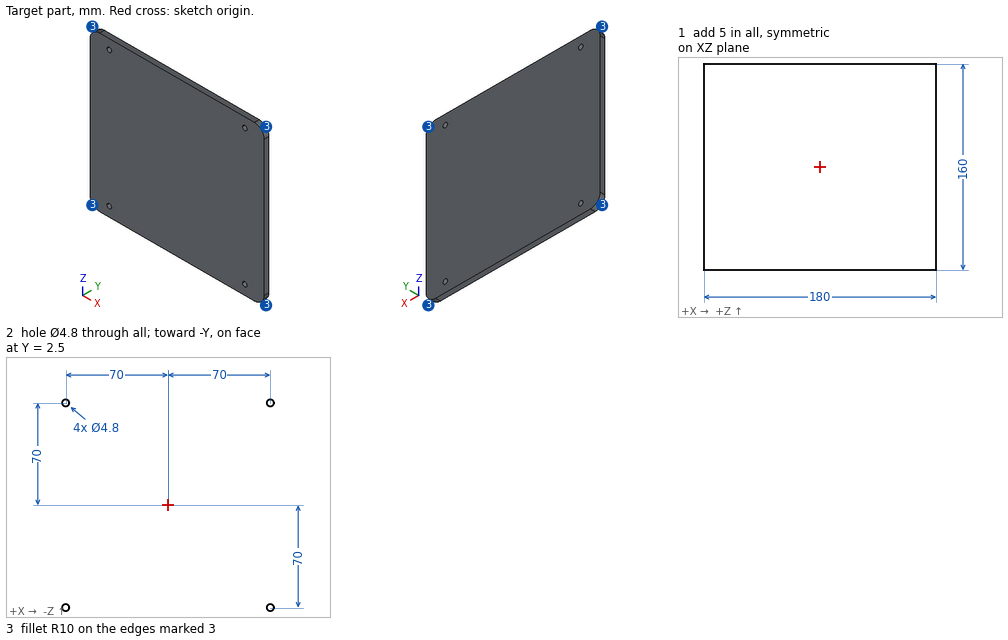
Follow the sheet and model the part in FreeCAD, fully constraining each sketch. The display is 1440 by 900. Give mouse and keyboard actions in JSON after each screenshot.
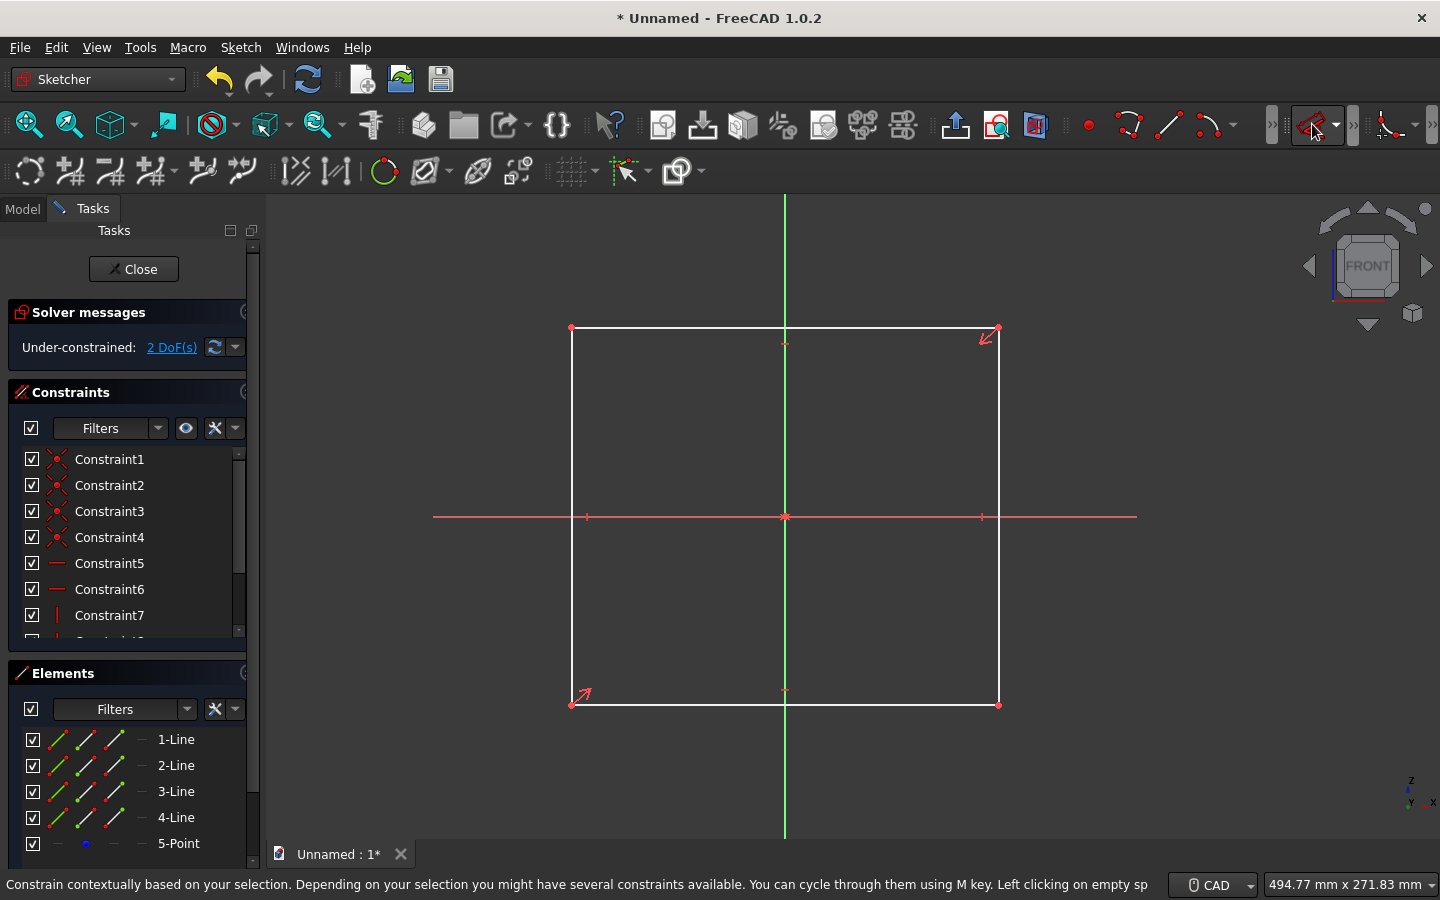
{"action": "left_click", "coordinate": [700, 705]}
{"action": "left_click", "coordinate": [687, 739]}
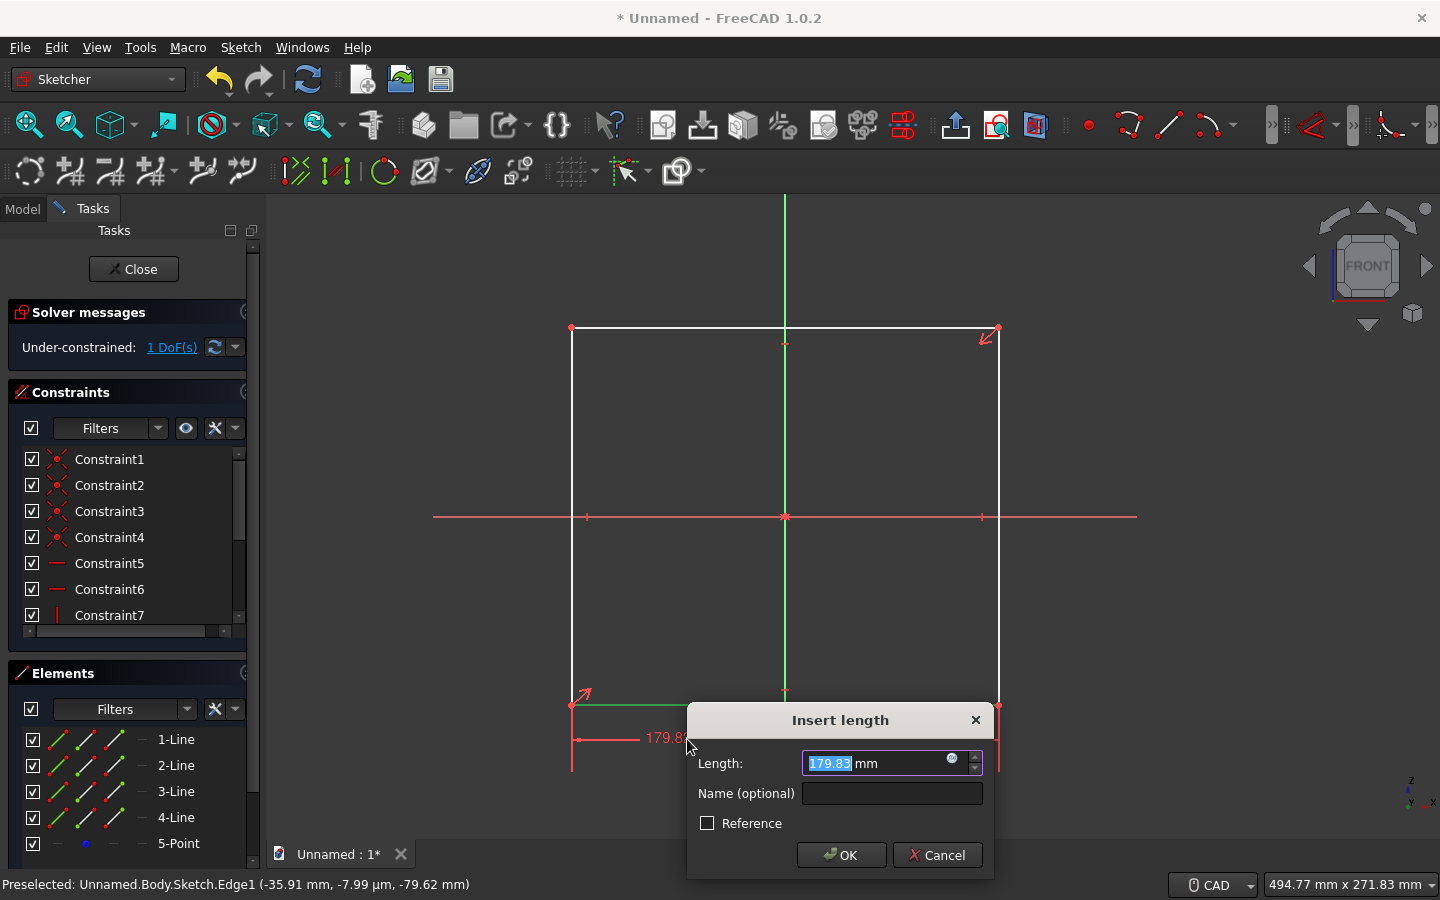
{"action": "type", "text": "180"}
{"action": "key", "text": "Return"}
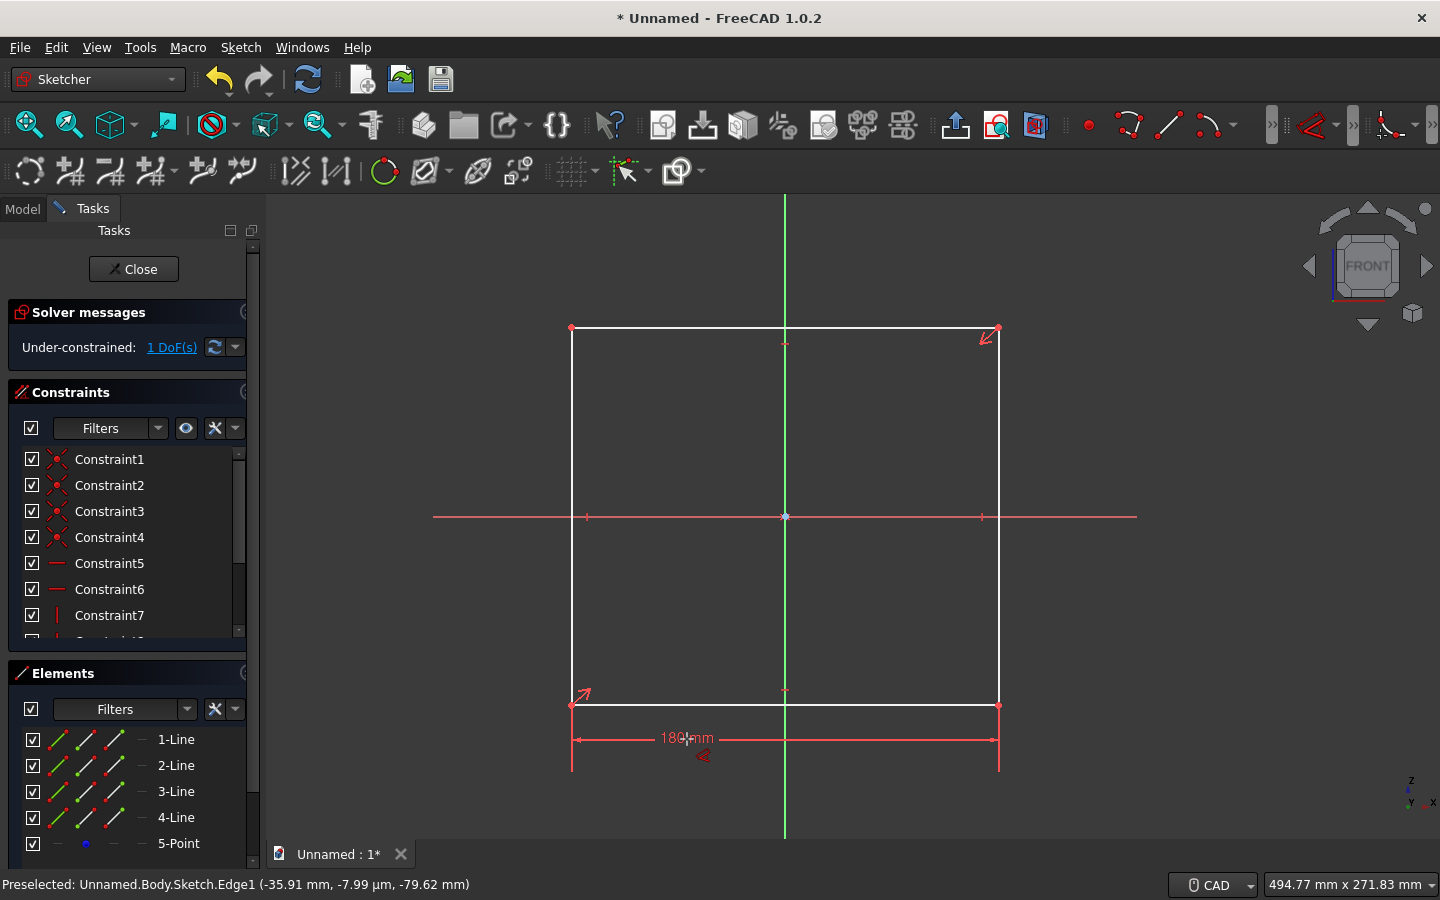
{"action": "left_click", "coordinate": [999, 592]}
{"action": "left_click", "coordinate": [1033, 430]}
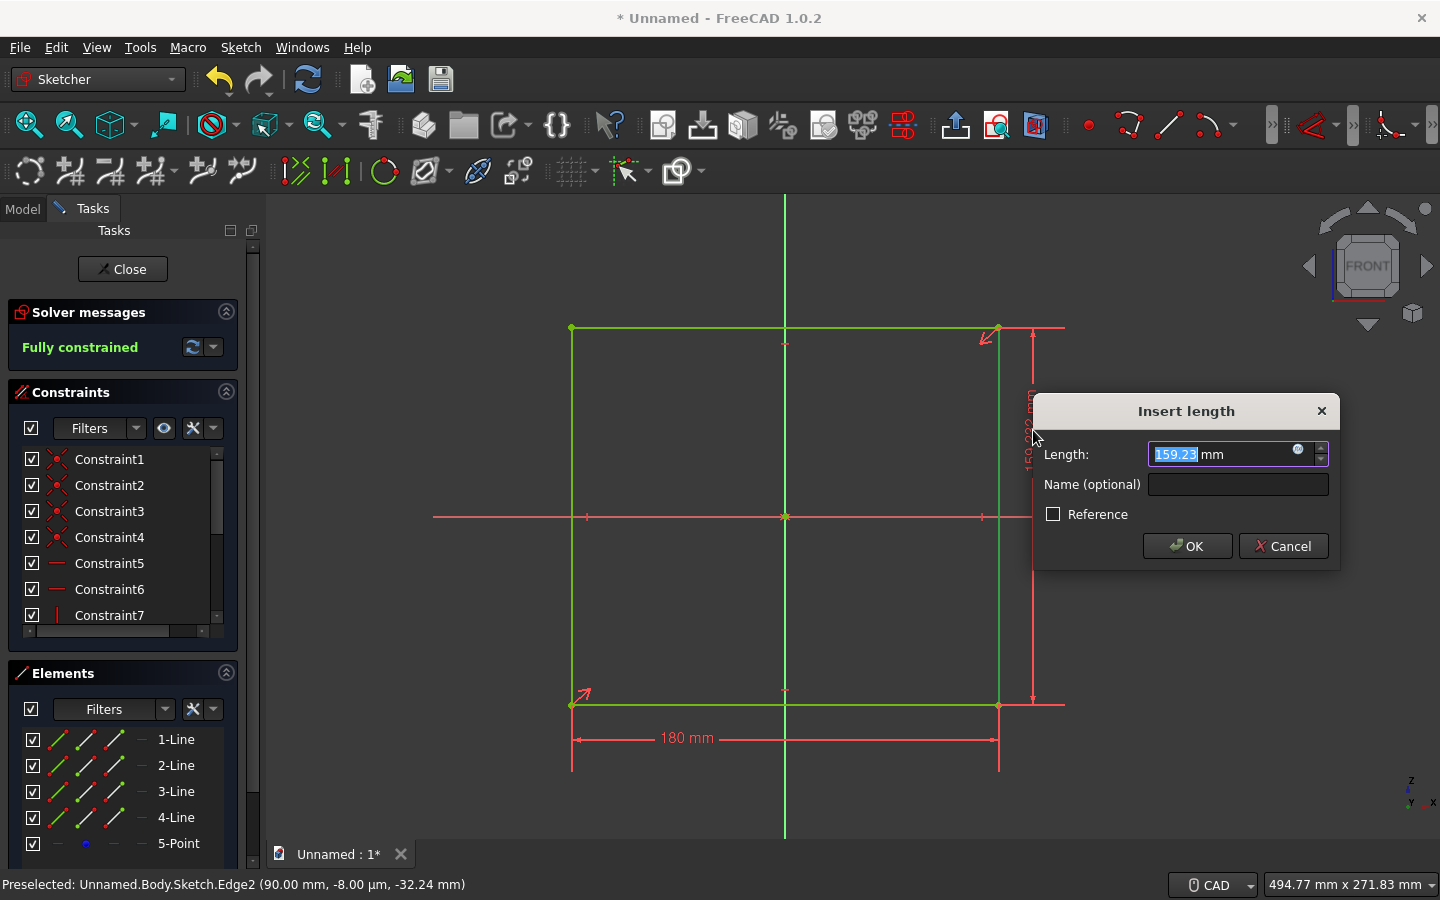
{"action": "type", "text": "160"}
{"action": "key", "text": "Return"}
{"action": "key", "text": "Escape"}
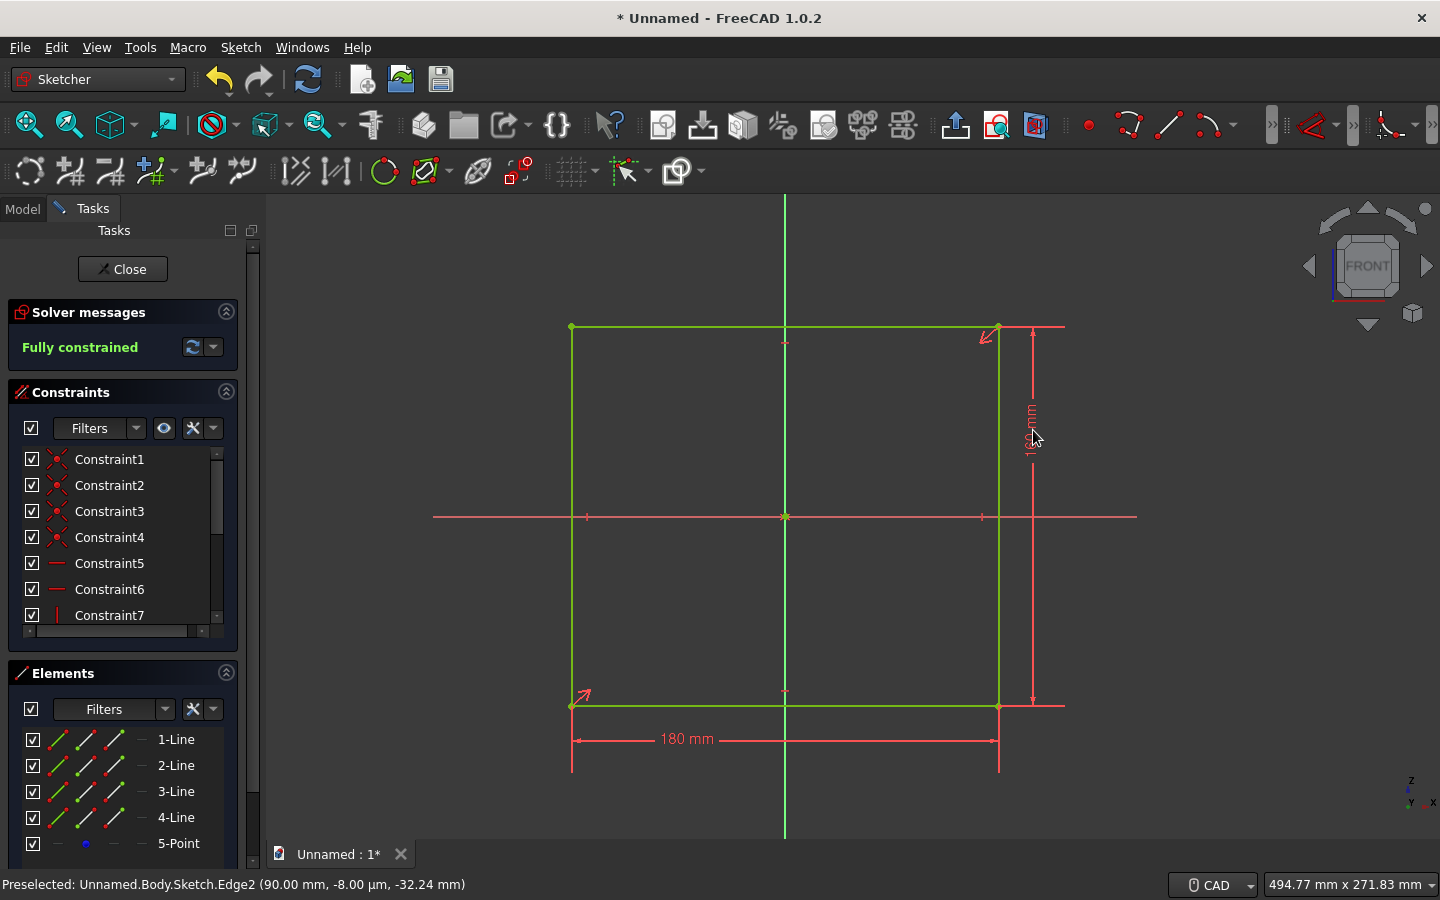
{"action": "left_click", "coordinate": [123, 269]}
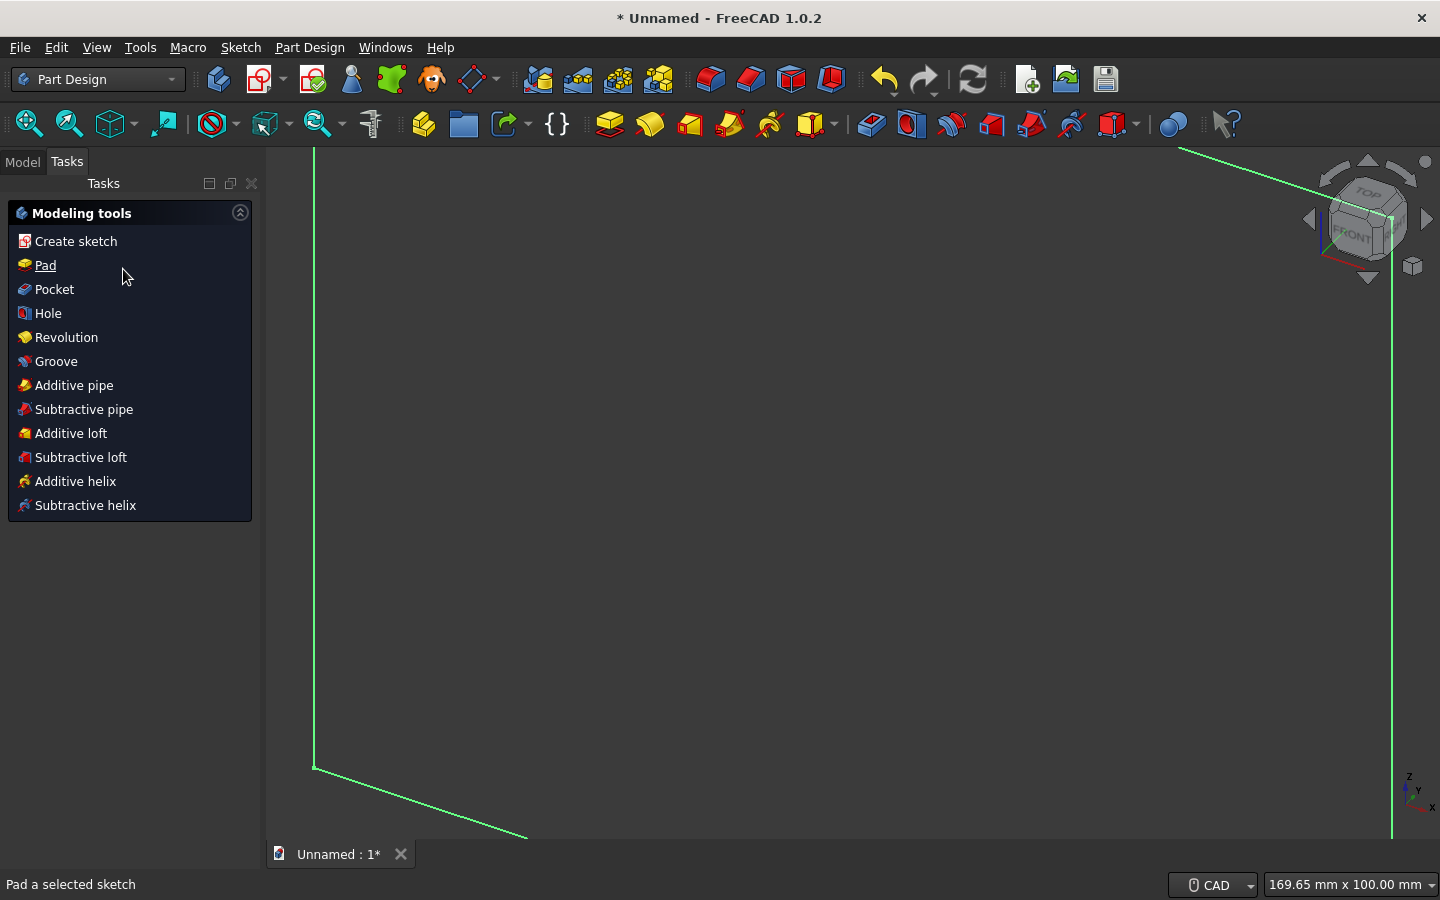
{"action": "left_click", "coordinate": [610, 124]}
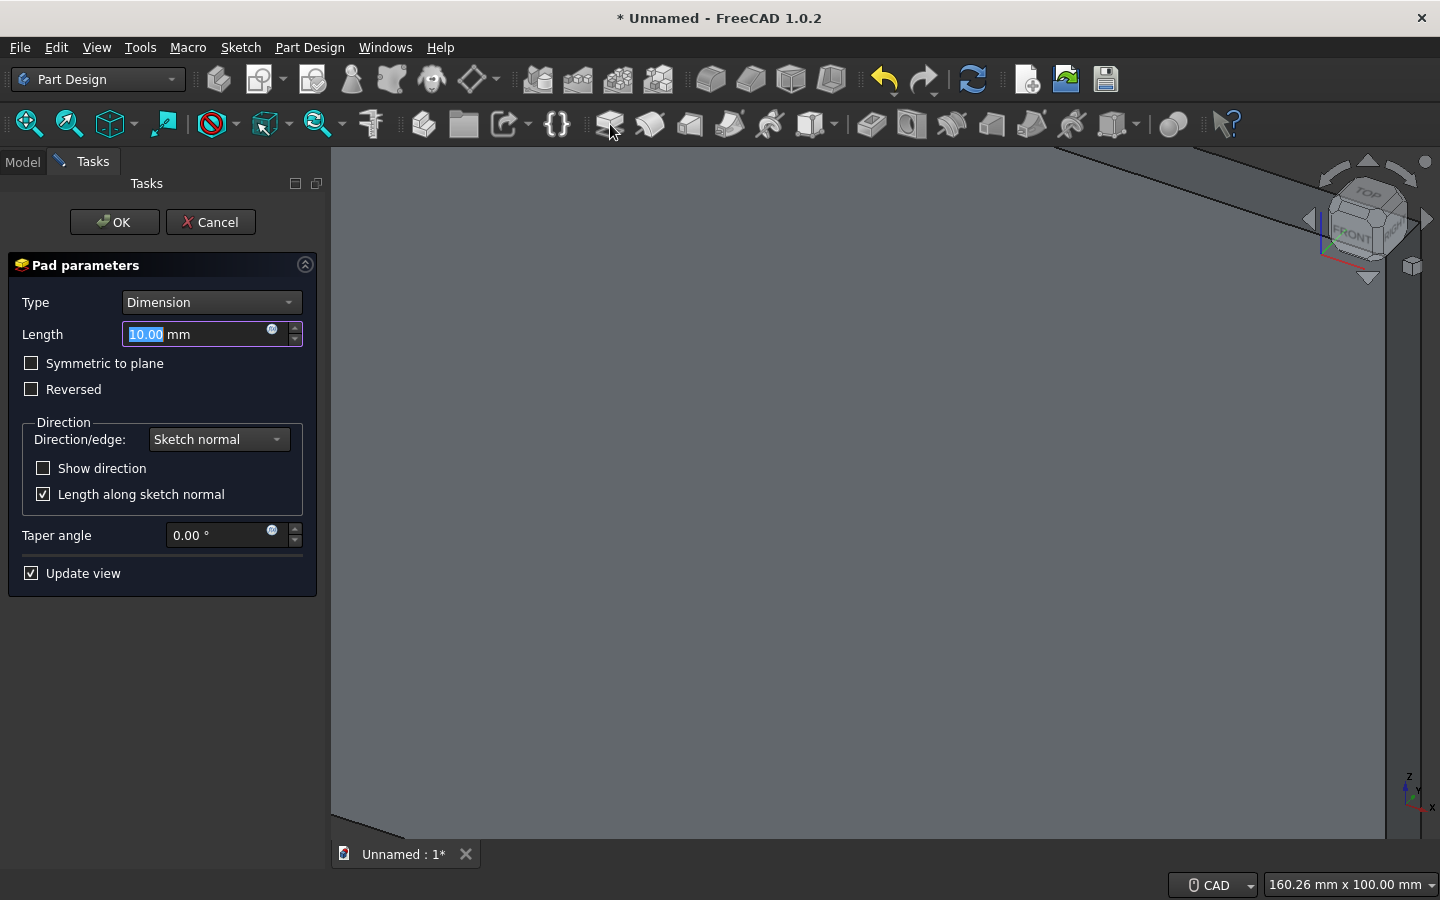
{"action": "type", "text": "5"}
{"action": "key", "text": "Tab"}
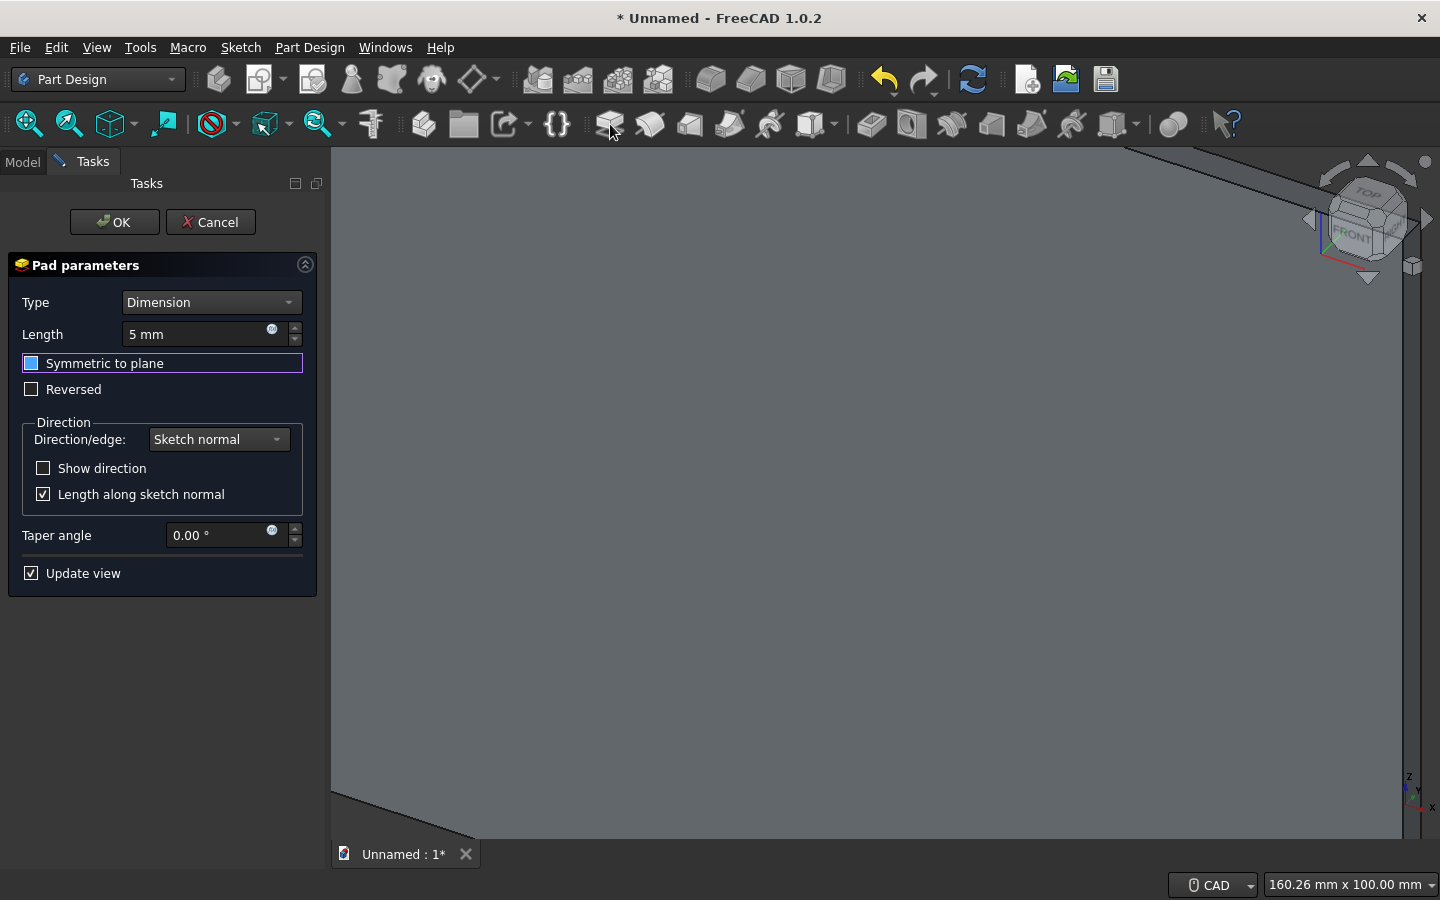
{"action": "left_click", "coordinate": [30, 363]}